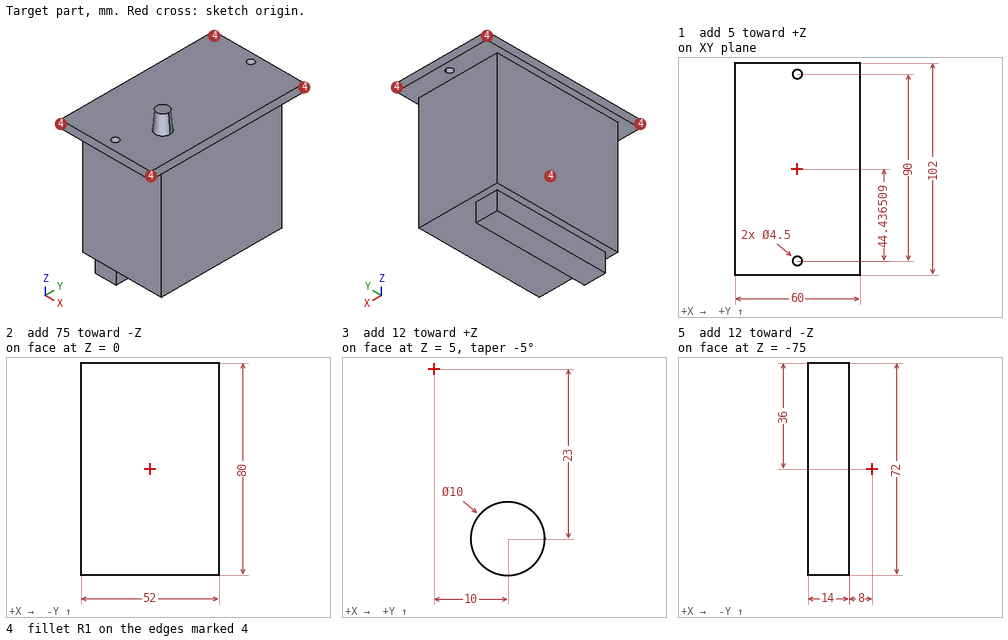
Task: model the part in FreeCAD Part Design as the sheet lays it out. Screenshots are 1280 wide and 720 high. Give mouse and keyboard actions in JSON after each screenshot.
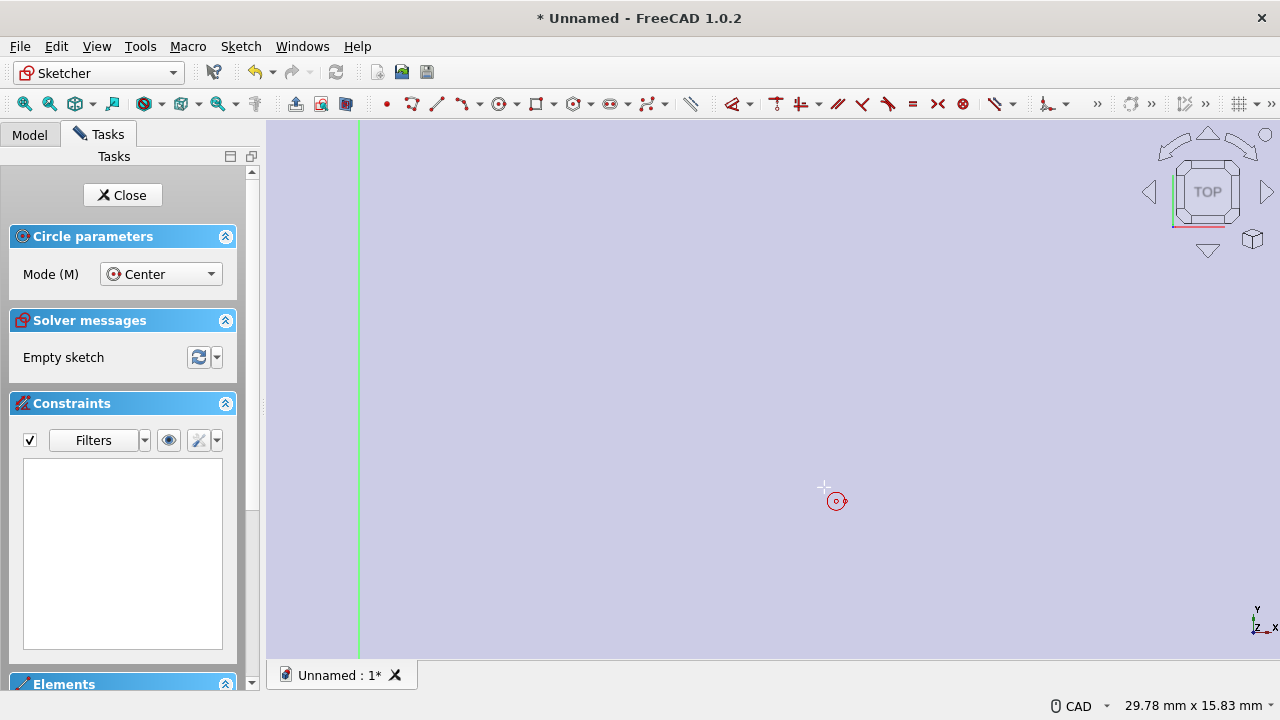
{"action": "left_click", "coordinate": [700, 385]}
{"action": "mouse_move", "coordinate": [820, 264]}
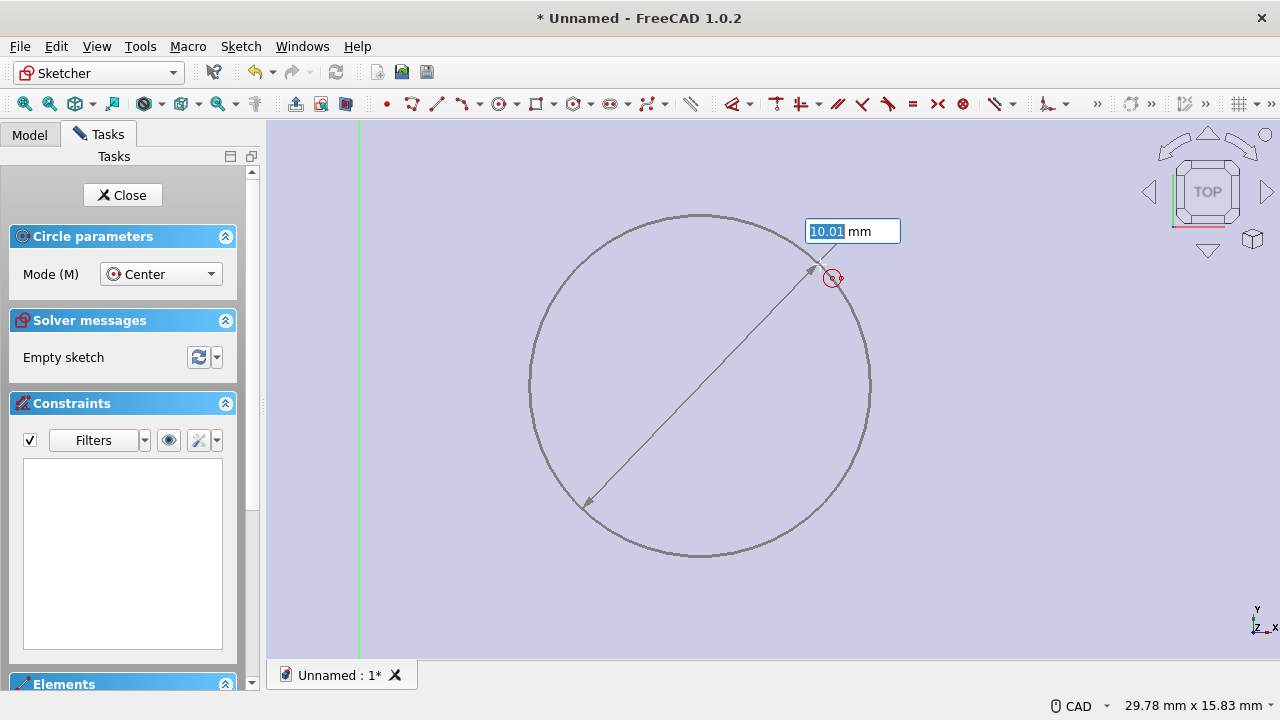
{"action": "type", "text": "10"}
{"action": "key", "text": "Return"}
{"action": "key", "text": "Escape"}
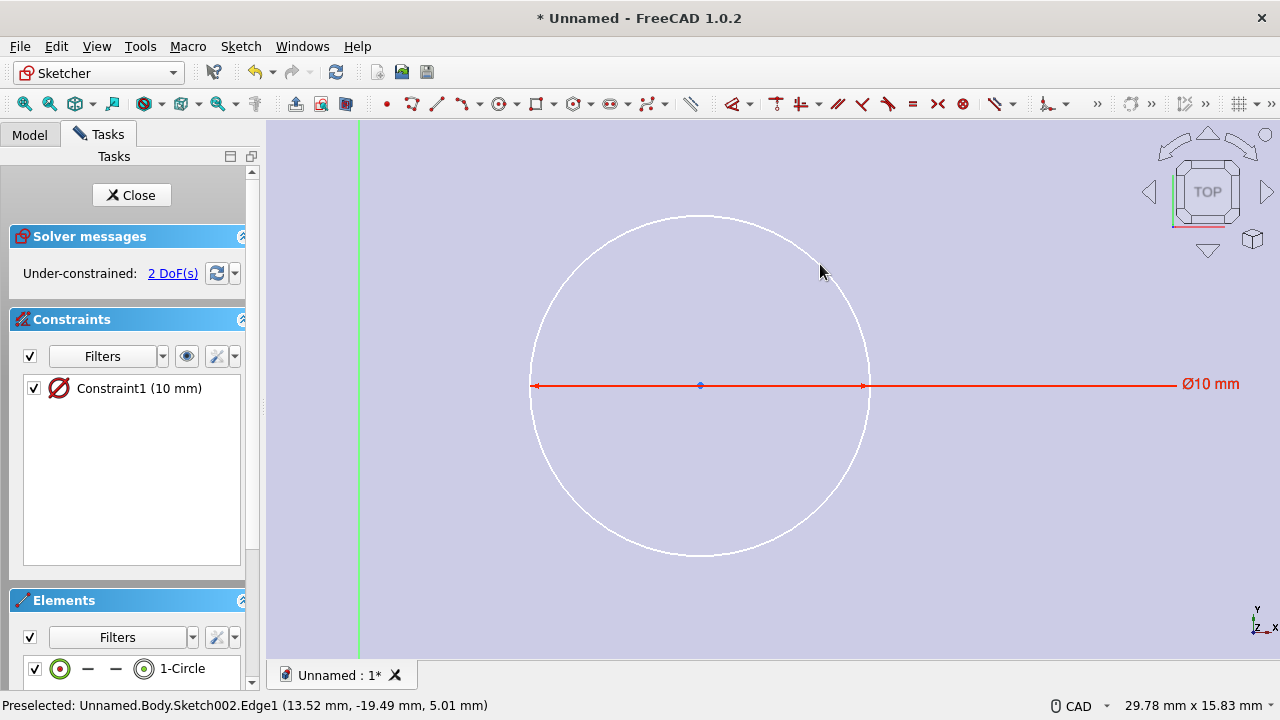
{"action": "left_click", "coordinate": [732, 104]}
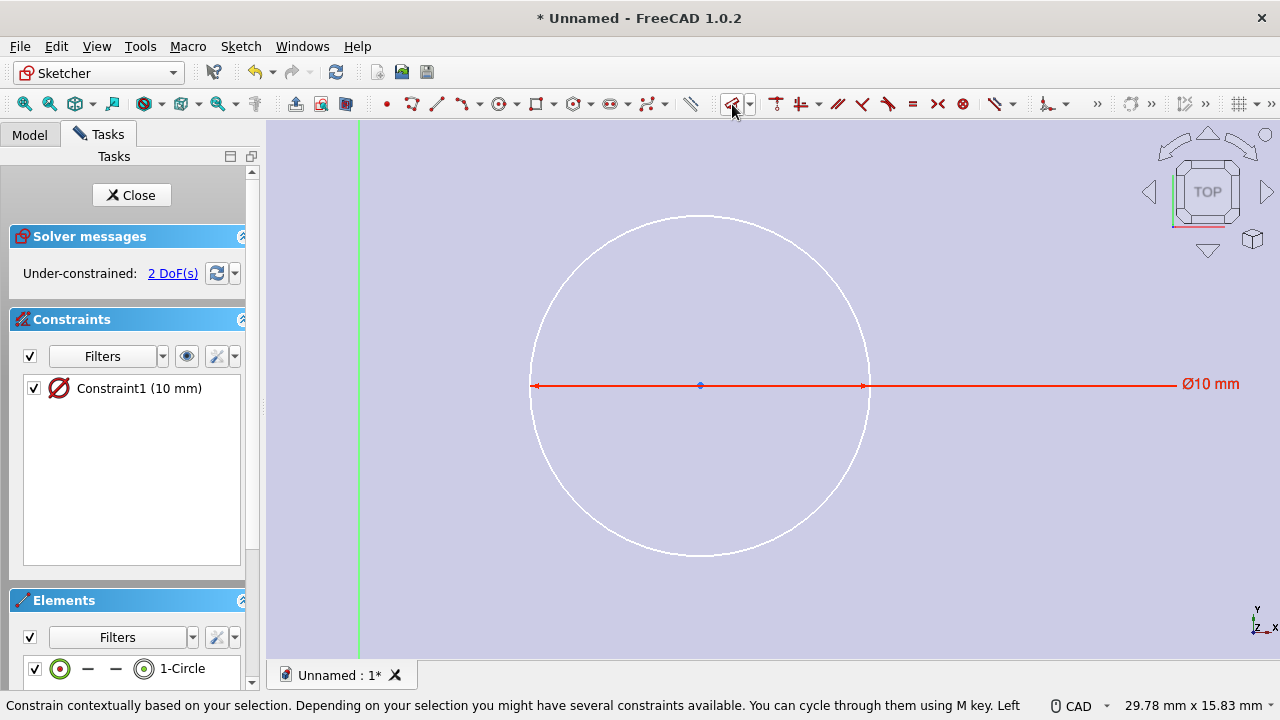
{"action": "left_click", "coordinate": [700, 386]}
{"action": "left_click", "coordinate": [451, 420]}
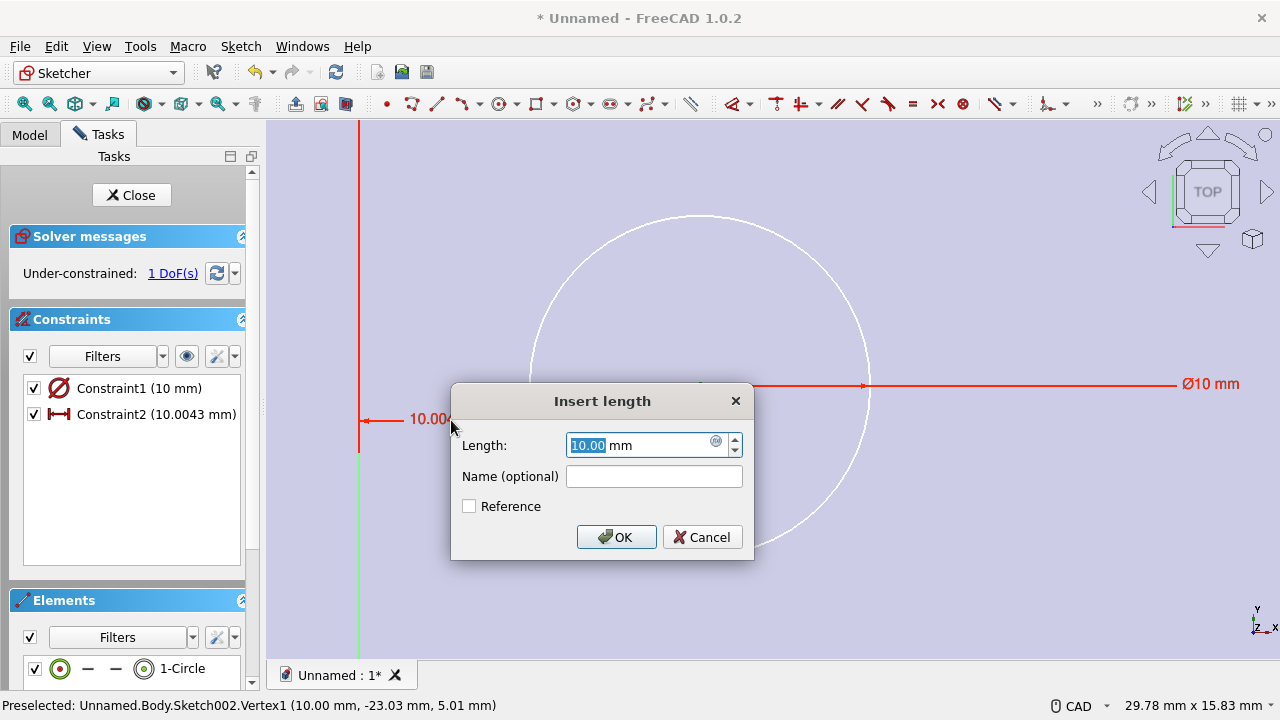
{"action": "type", "text": "10"}
{"action": "key", "text": "Return"}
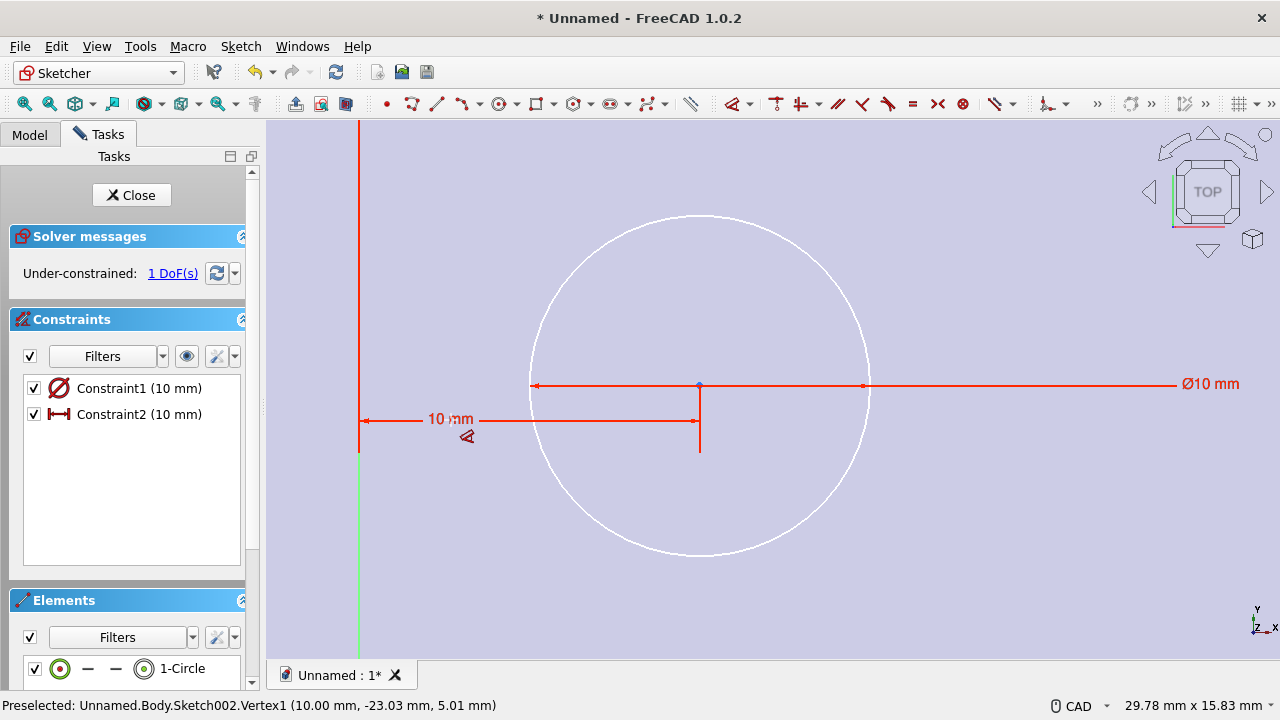
{"action": "left_click", "coordinate": [700, 386]}
{"action": "left_click", "coordinate": [325, 267]}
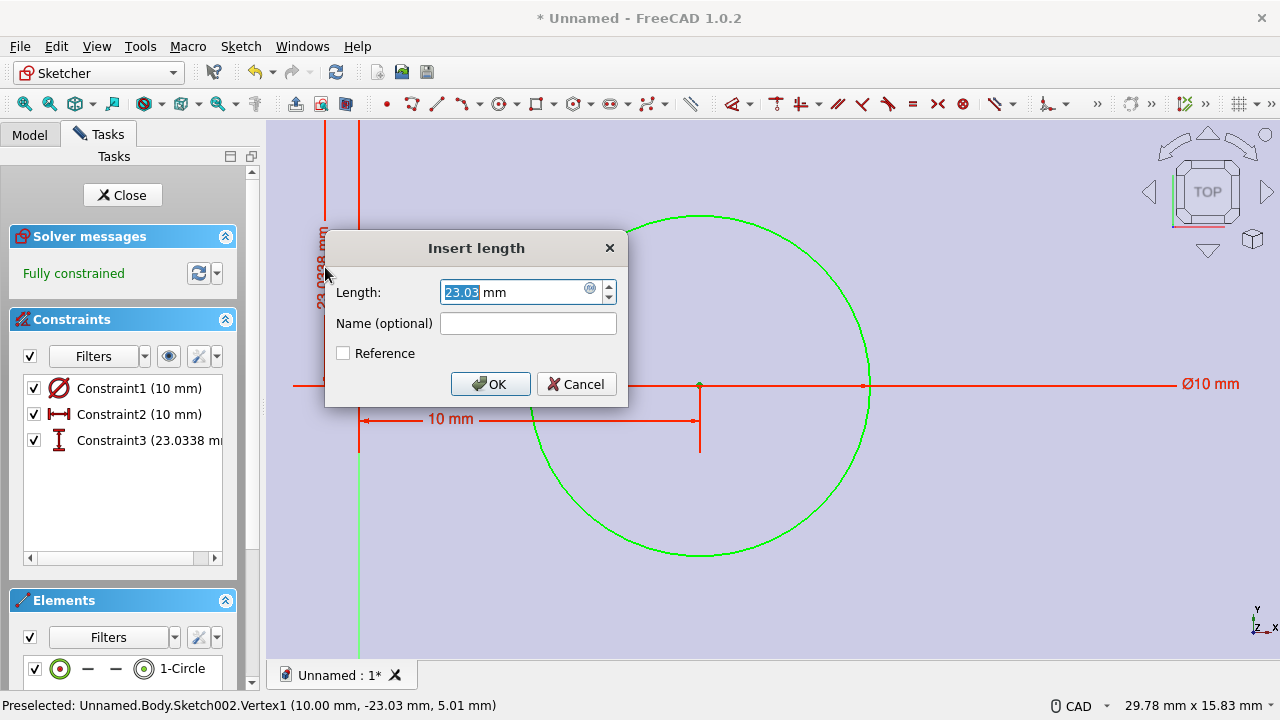
{"action": "type", "text": "23"}
{"action": "key", "text": "Return"}
{"action": "key", "text": "Escape"}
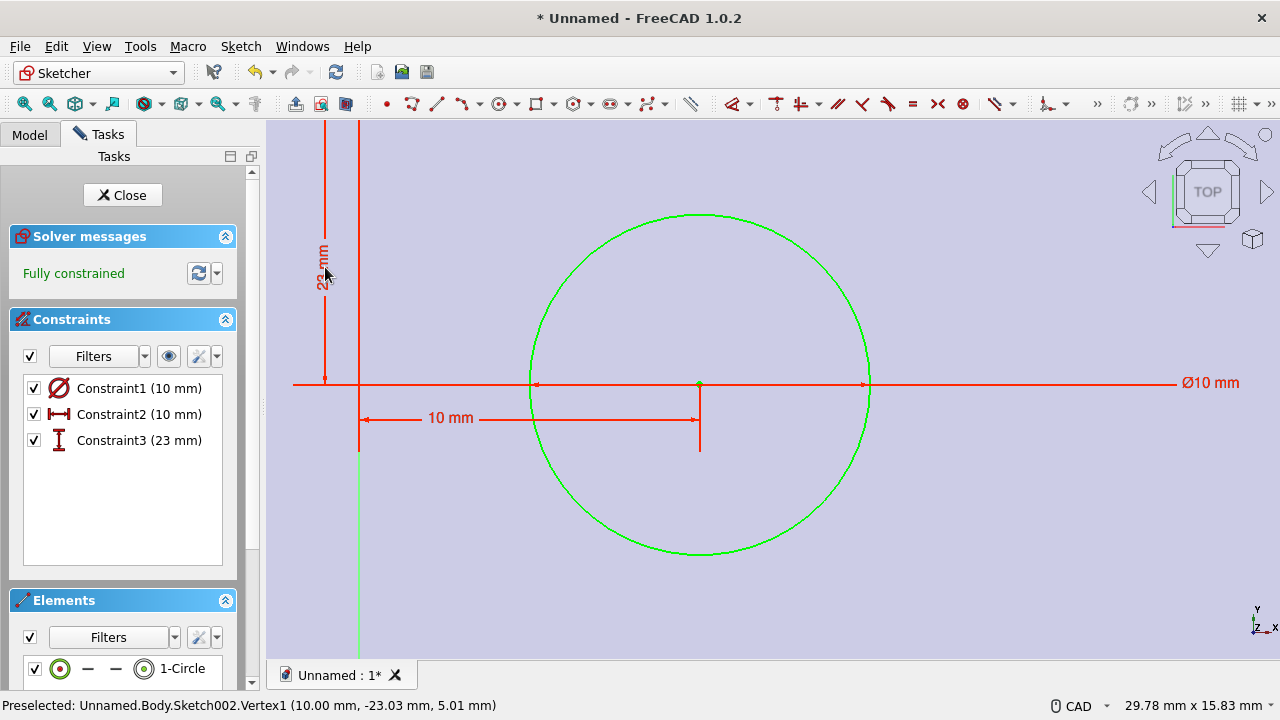
{"action": "left_click", "coordinate": [123, 195]}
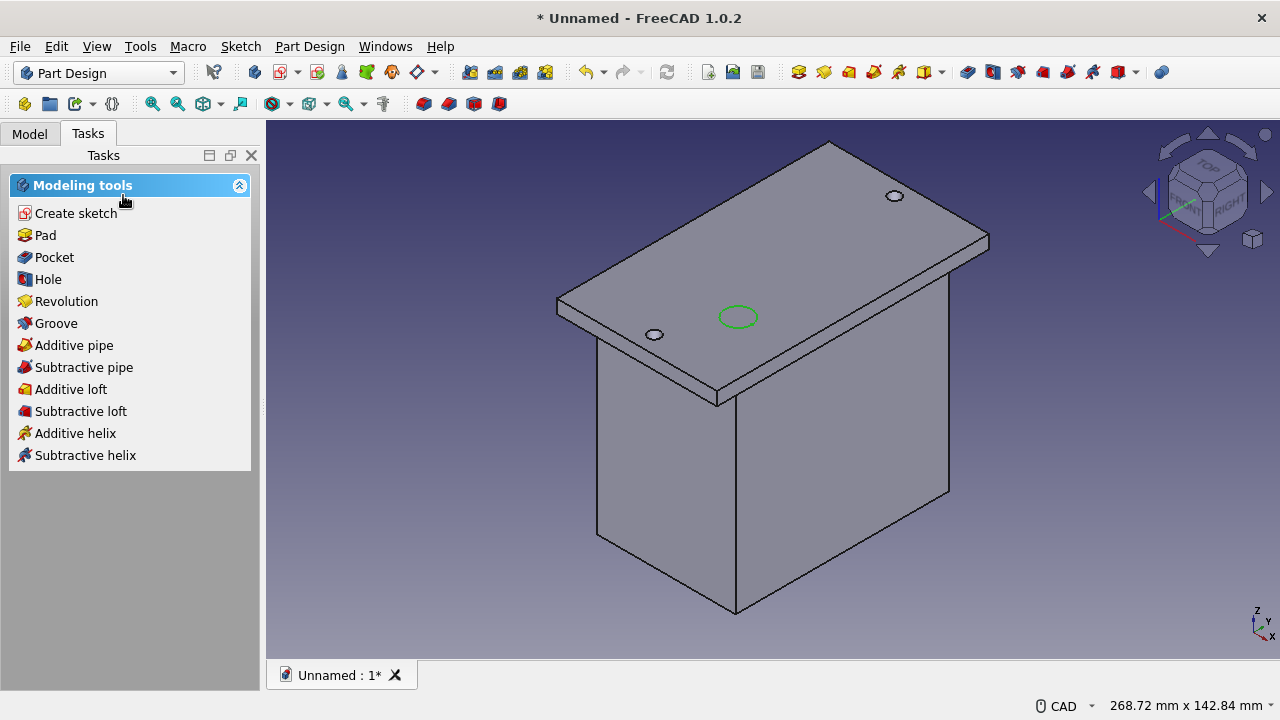
{"action": "left_click", "coordinate": [799, 72]}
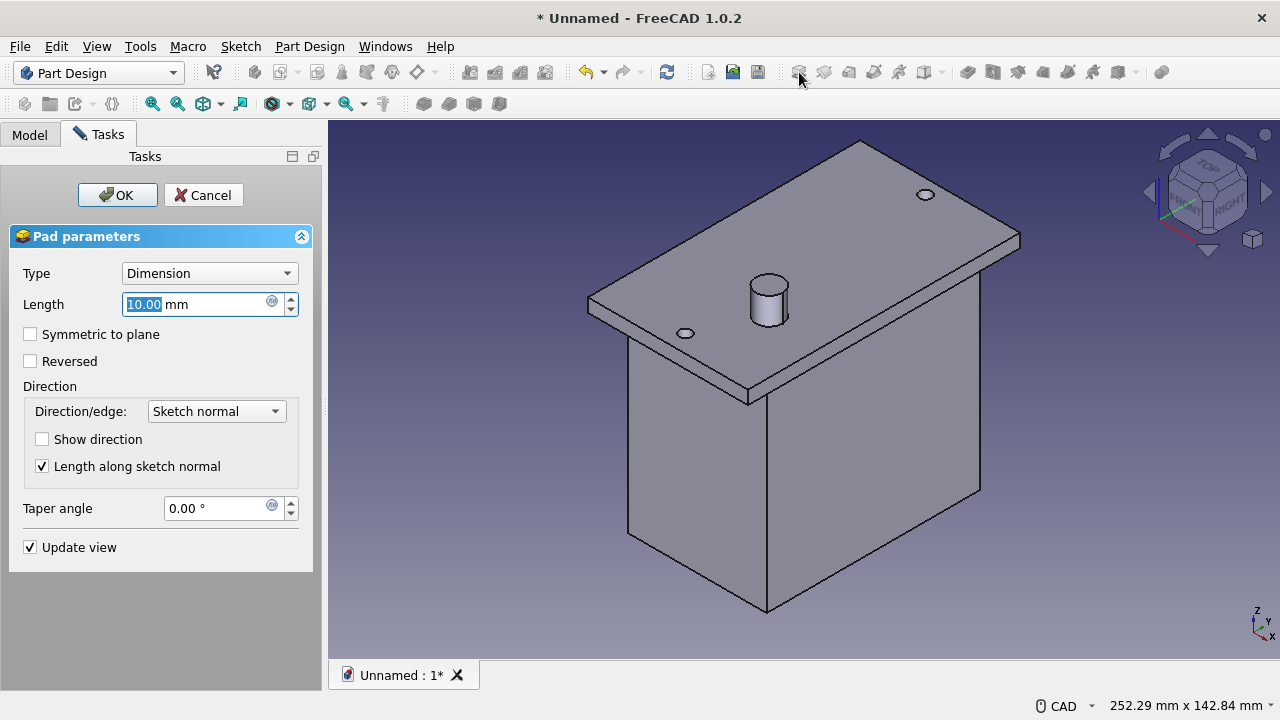
{"action": "type", "text": "12"}
{"action": "key", "text": "Tab"}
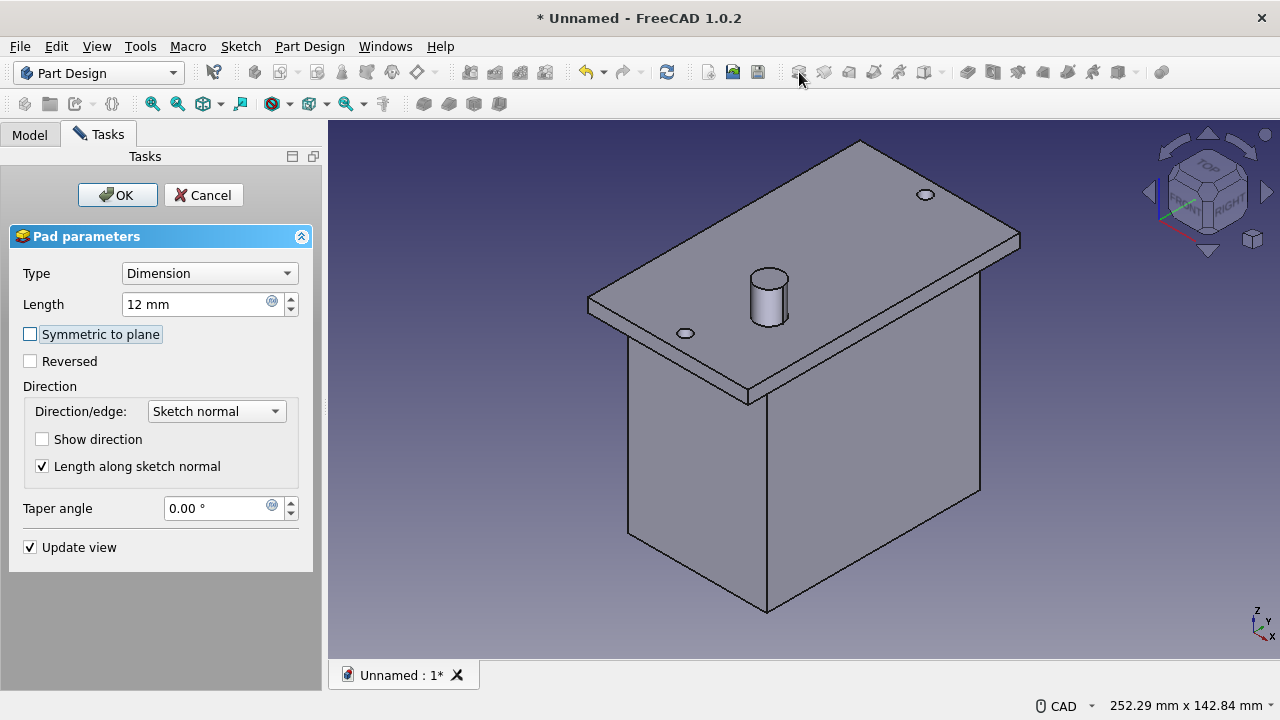
{"action": "triple_click", "coordinate": [224, 508]}